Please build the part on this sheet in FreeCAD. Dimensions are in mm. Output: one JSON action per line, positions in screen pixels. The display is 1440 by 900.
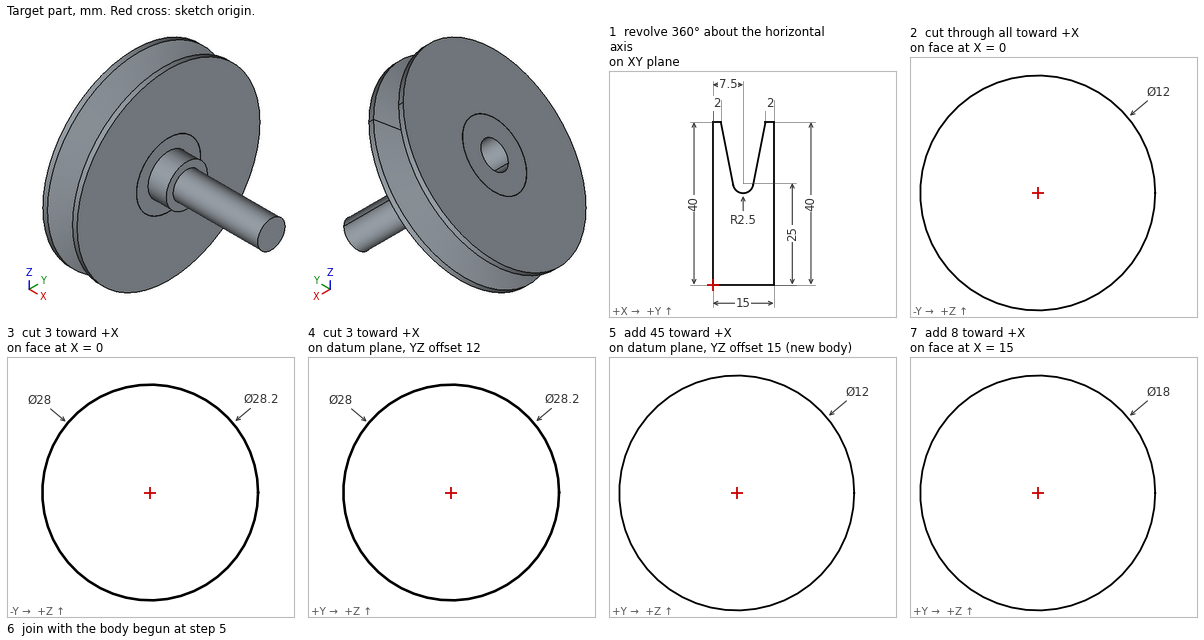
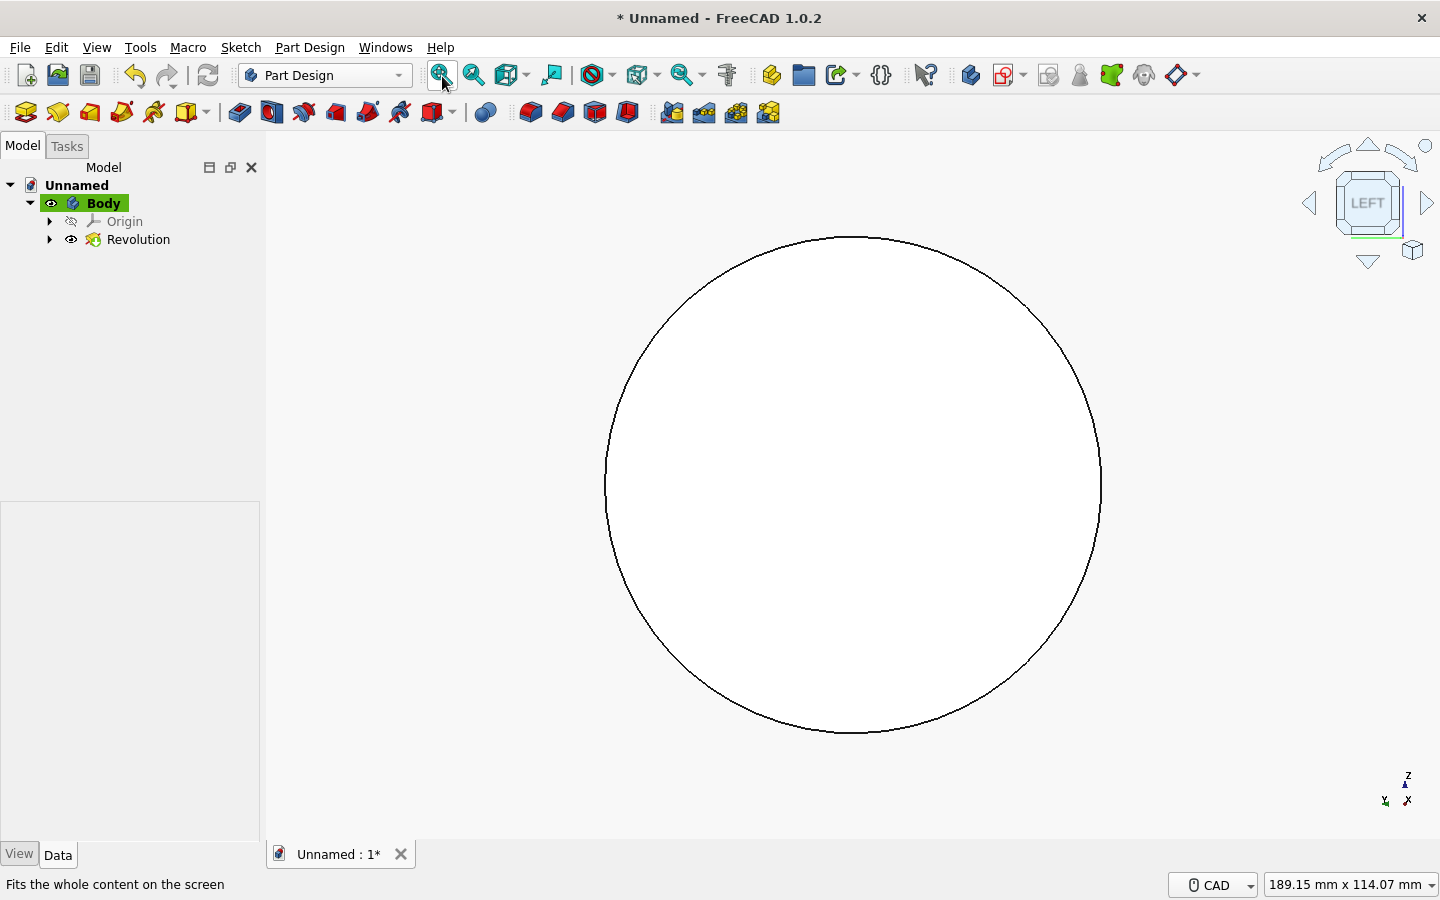
{"action": "left_click", "coordinate": [853, 484]}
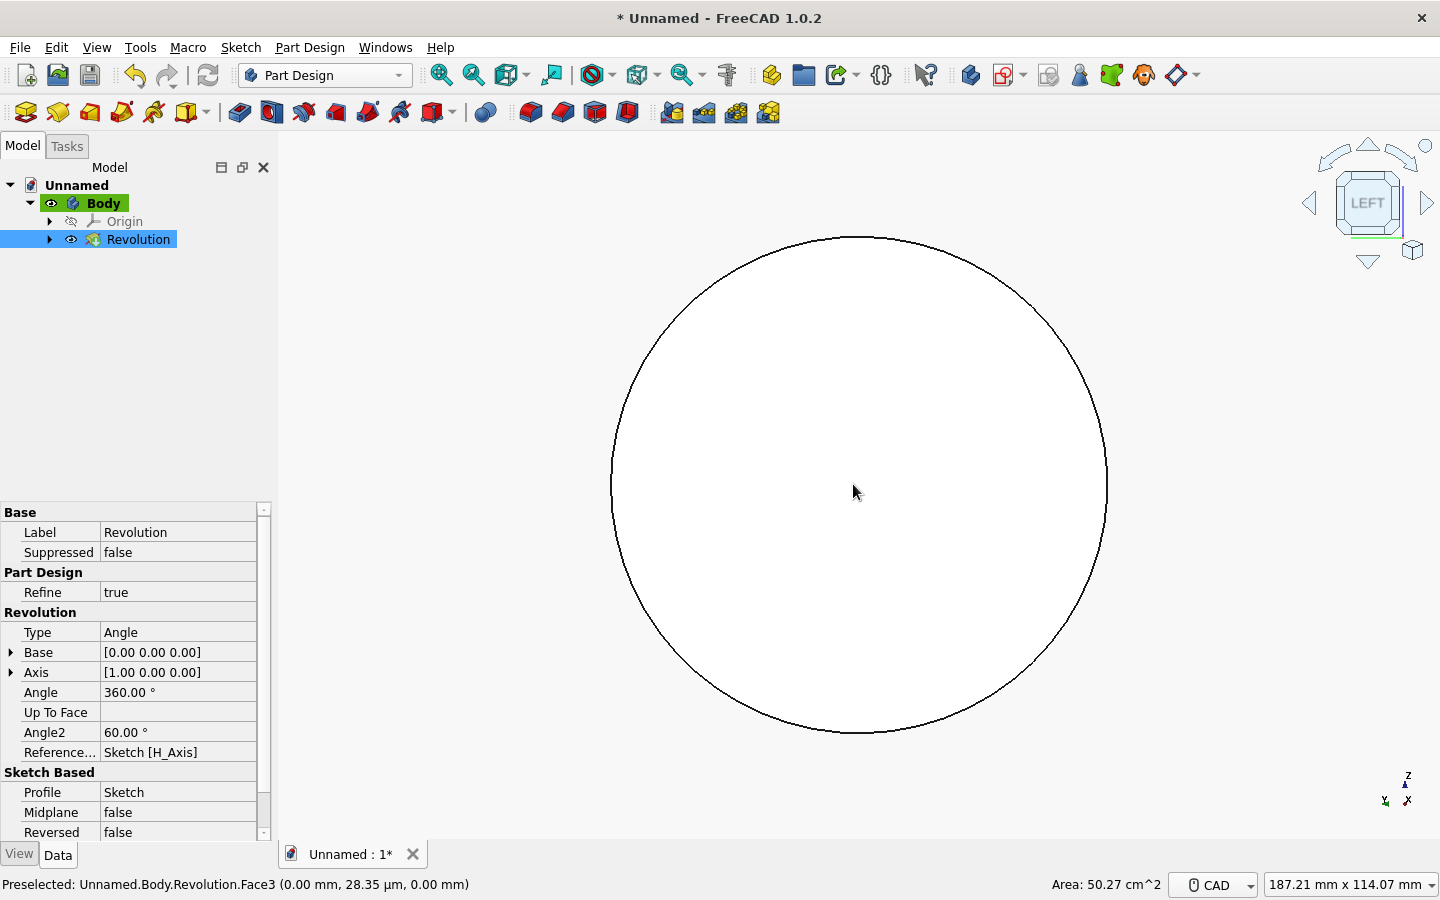
{"action": "left_click", "coordinate": [1004, 76]}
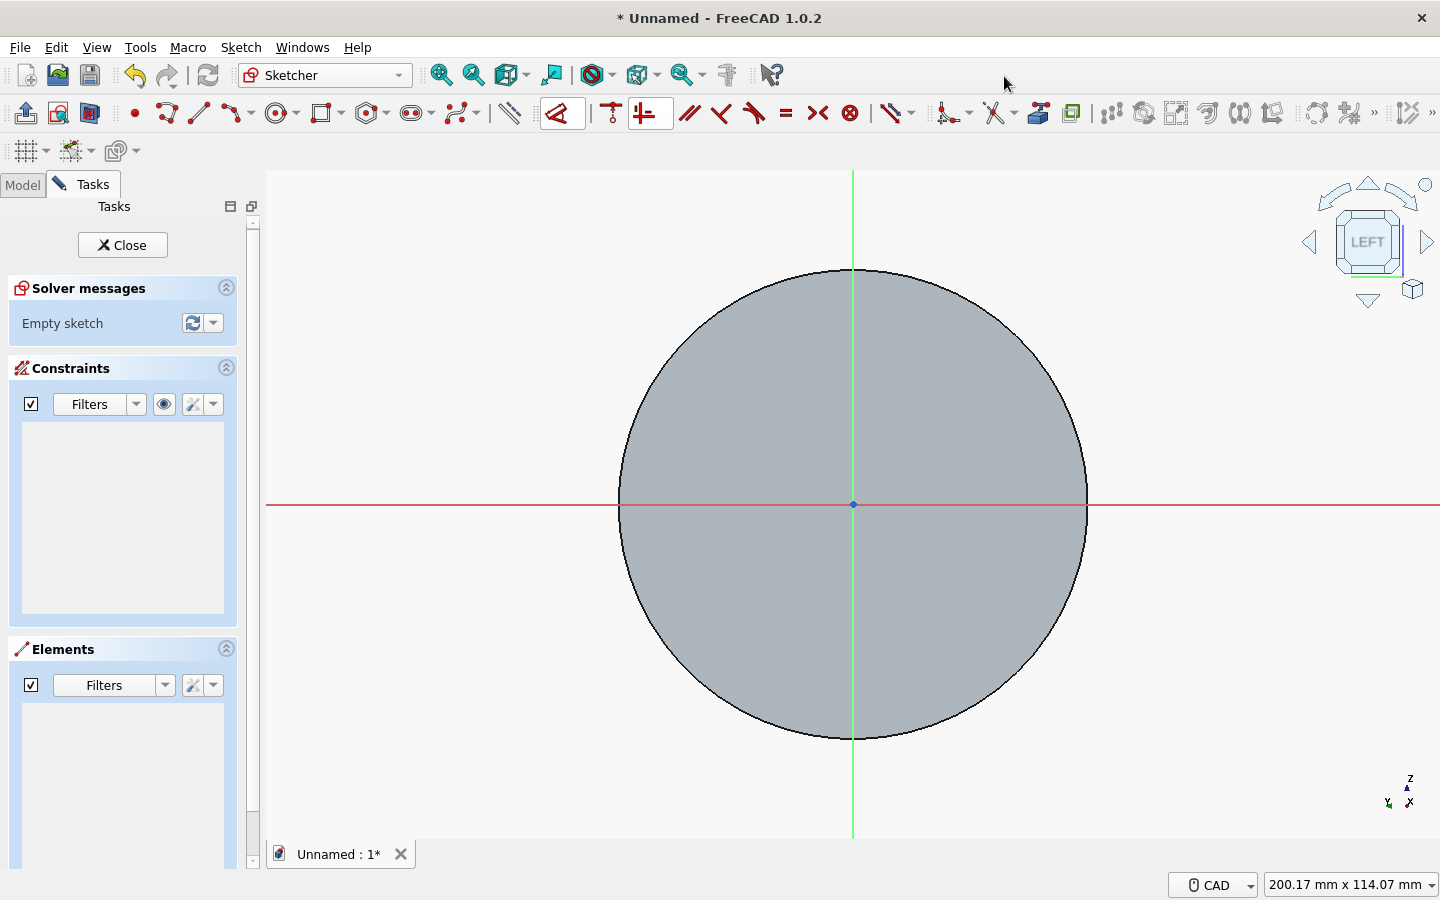
{"action": "scroll", "coordinate": [867, 505], "scroll_direction": "up", "scroll_amount": 9}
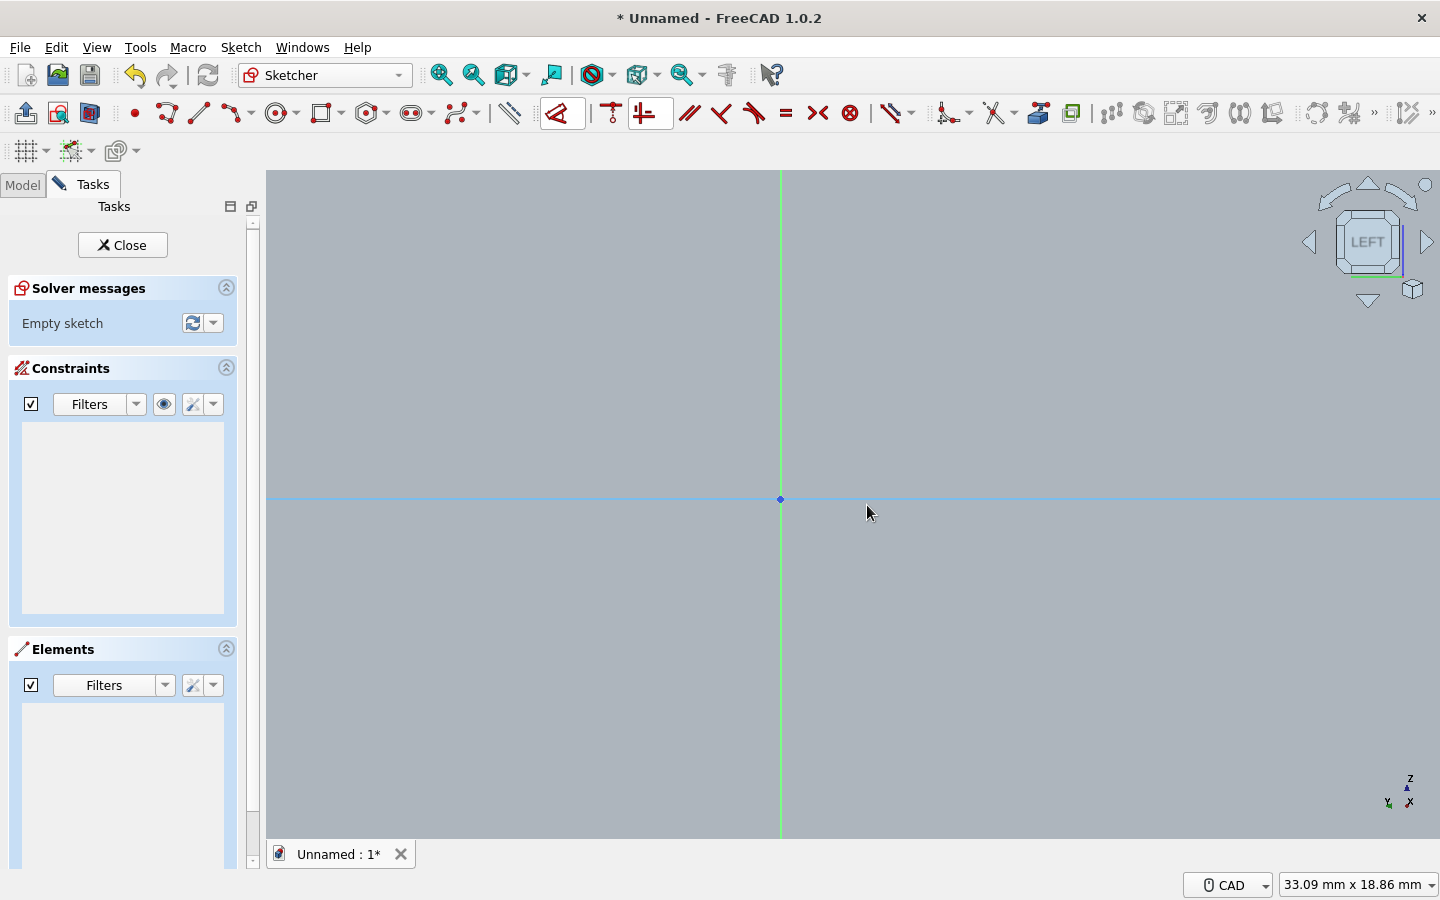
{"action": "key", "text": "g c"}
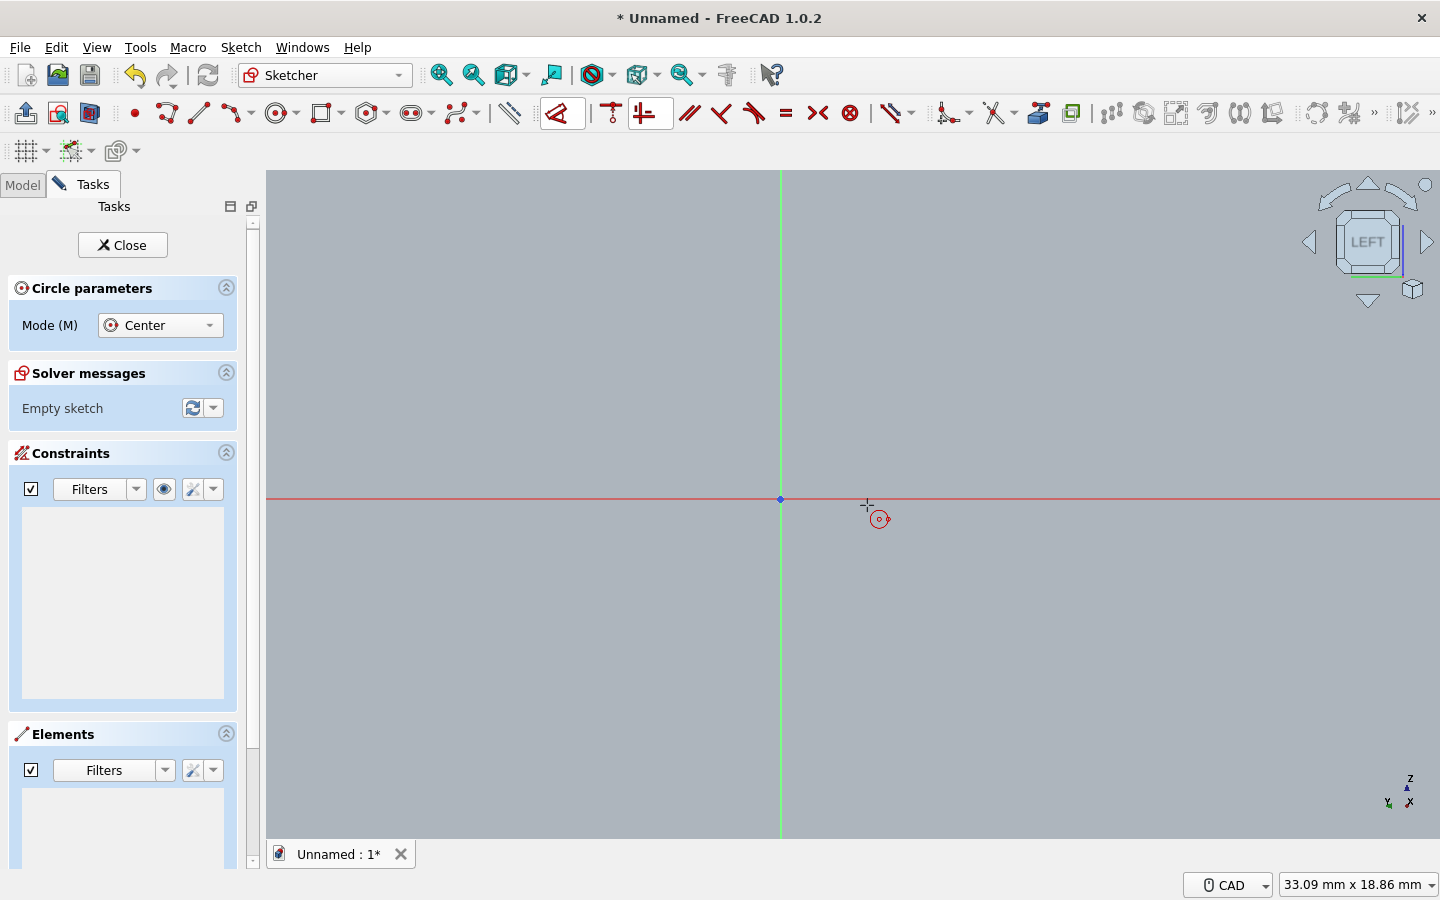
{"action": "left_click", "coordinate": [781, 499]}
{"action": "mouse_move", "coordinate": [931, 349]}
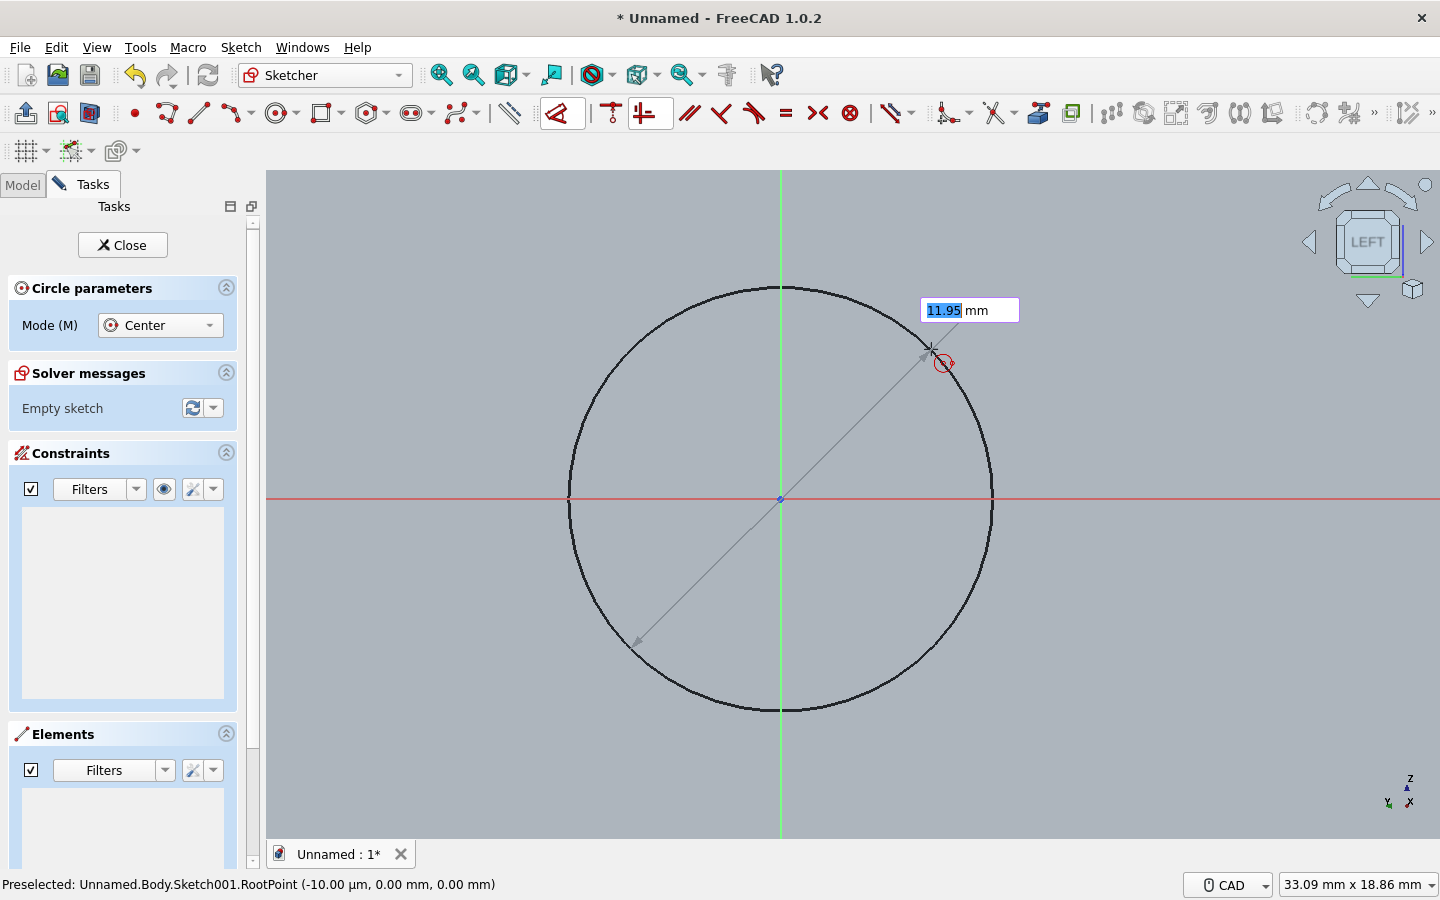
{"action": "type", "text": "12"}
{"action": "key", "text": "Return"}
{"action": "key", "text": "Escape"}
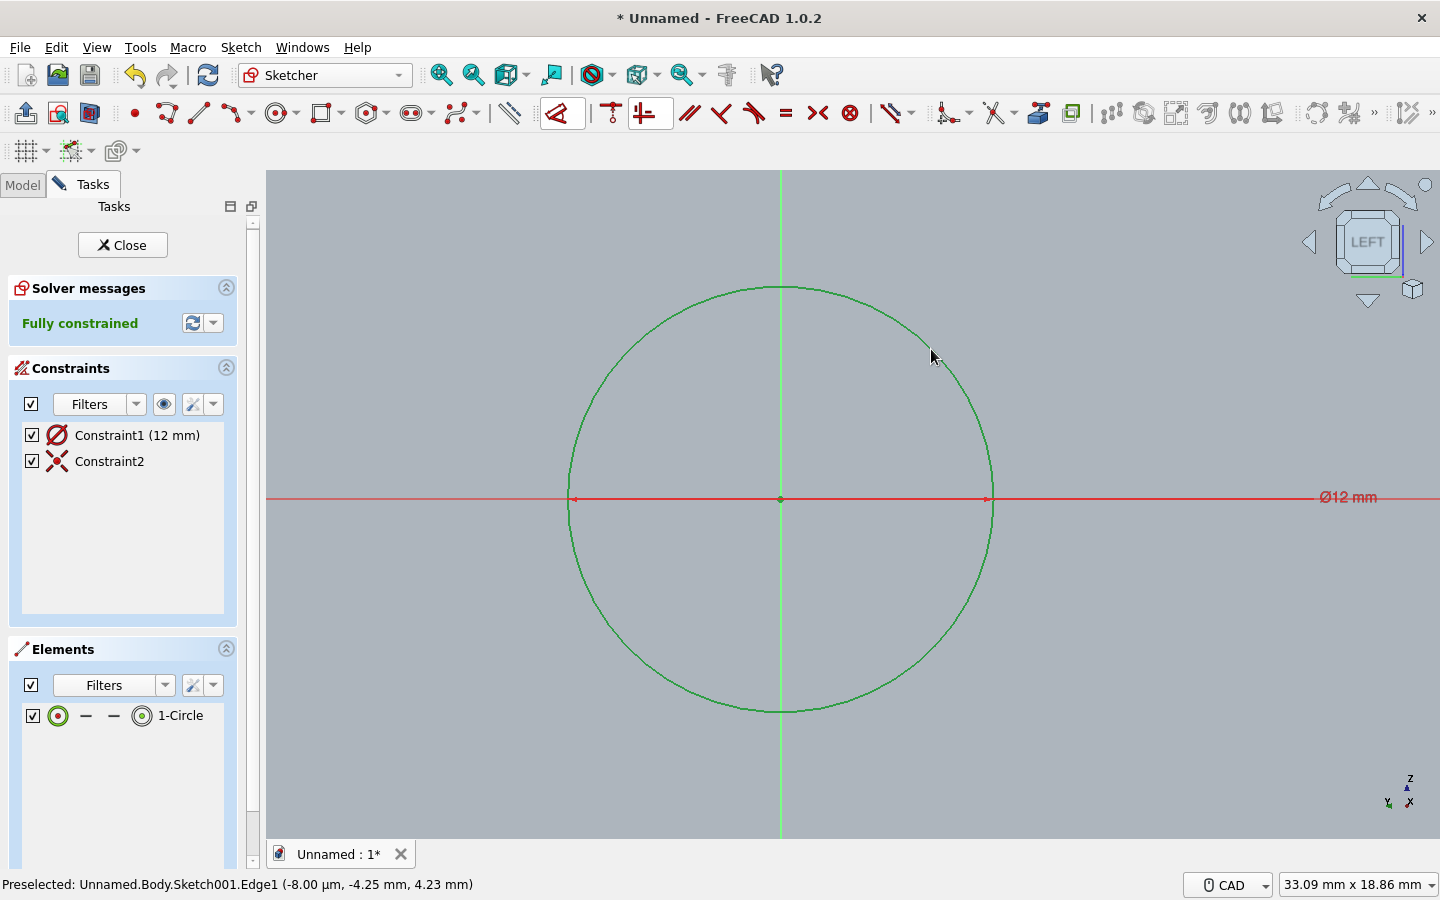
{"action": "left_click", "coordinate": [123, 245]}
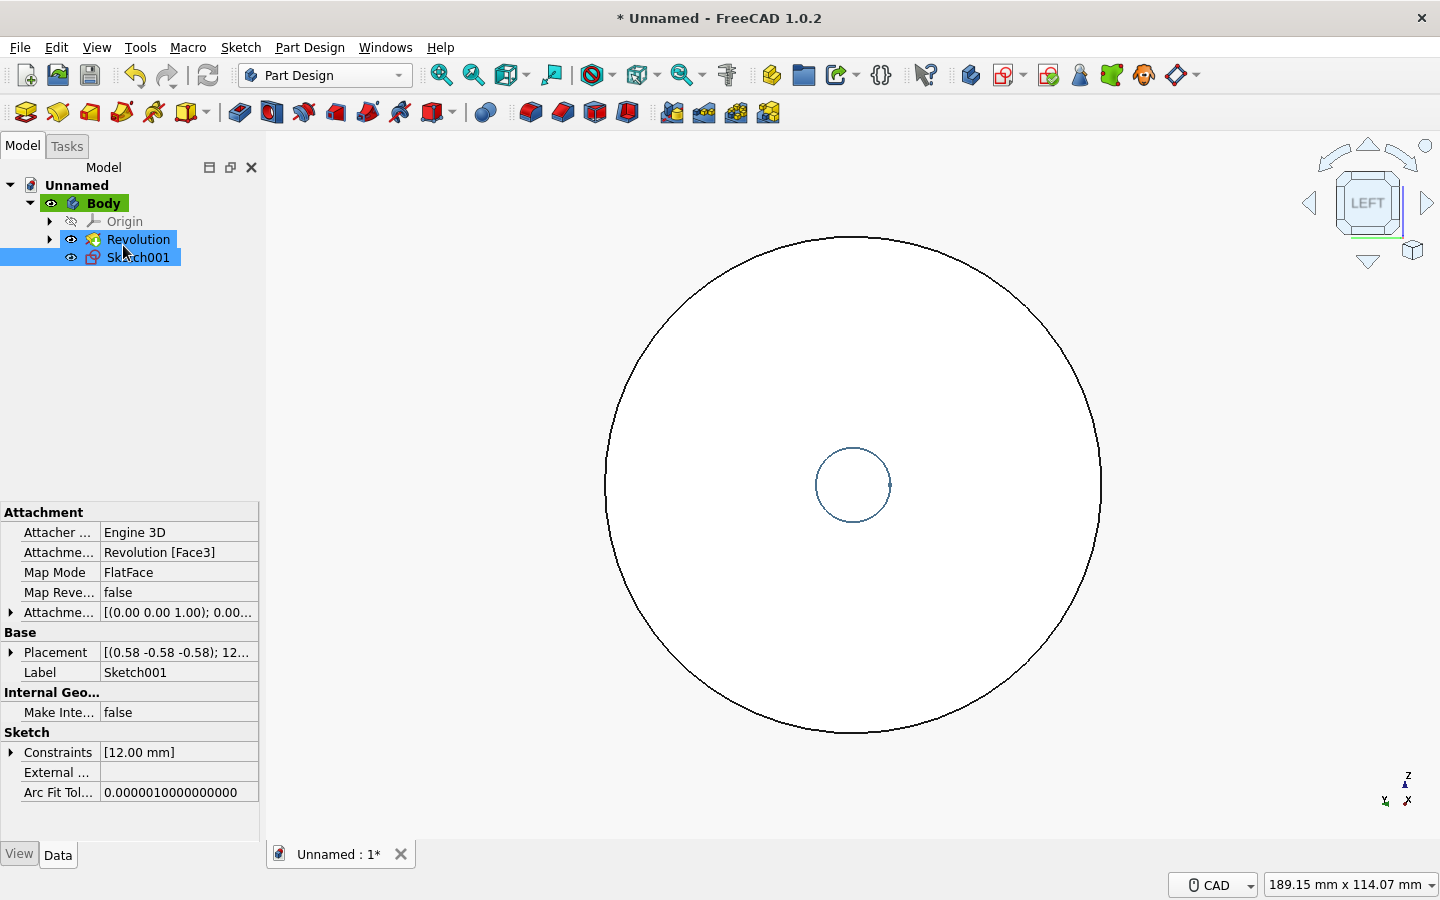
{"action": "left_click", "coordinate": [240, 112]}